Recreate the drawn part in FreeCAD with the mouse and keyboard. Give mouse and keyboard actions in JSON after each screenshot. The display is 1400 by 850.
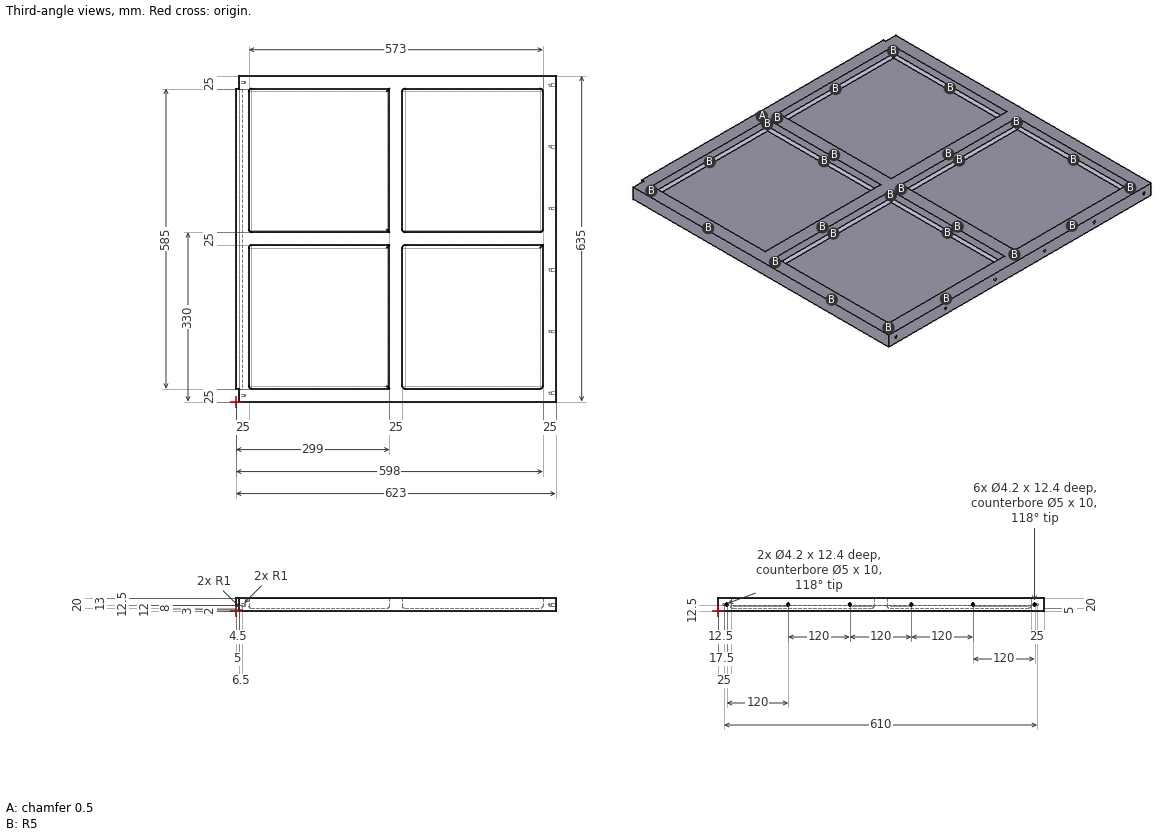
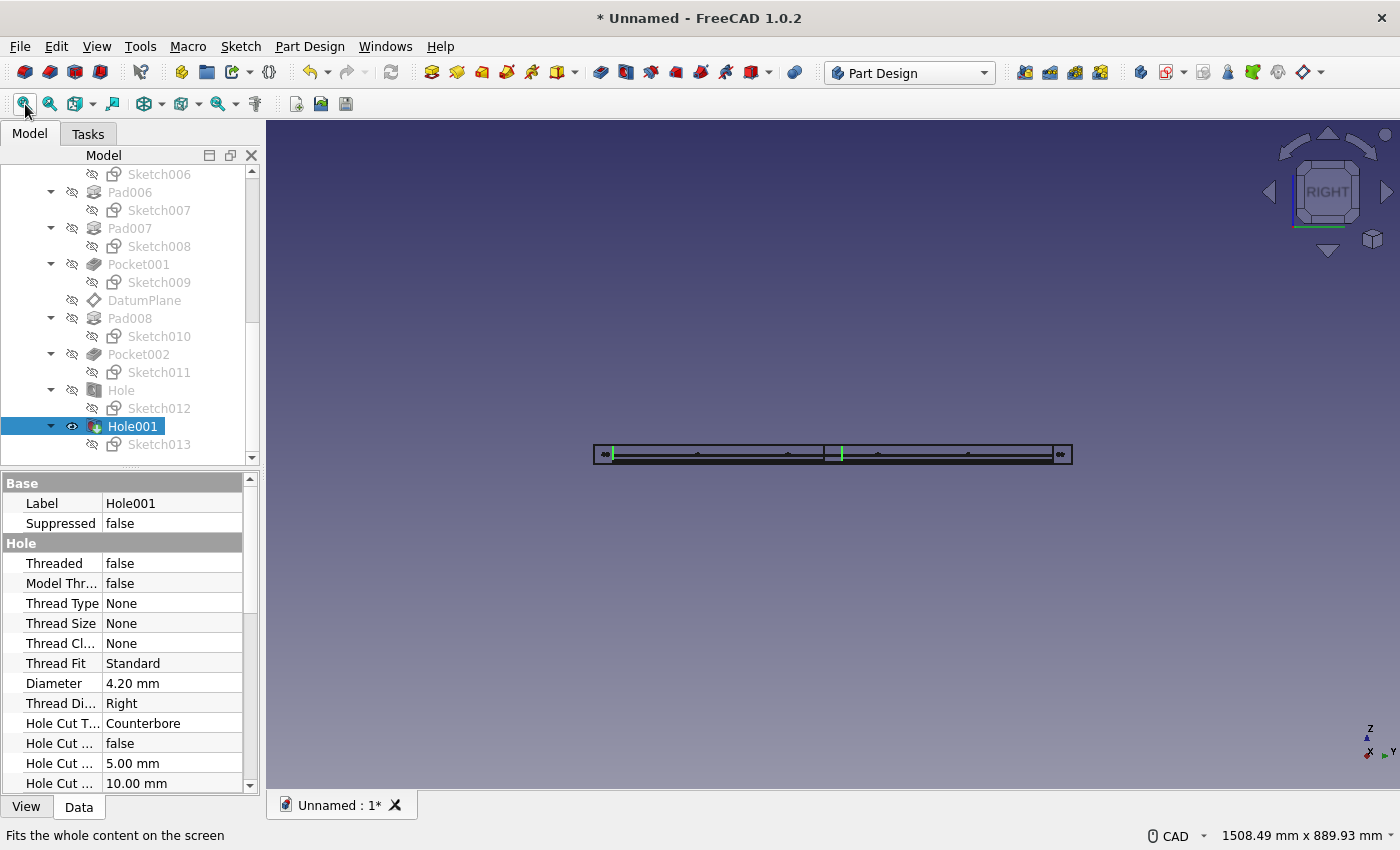
{"action": "left_click", "coordinate": [25, 104]}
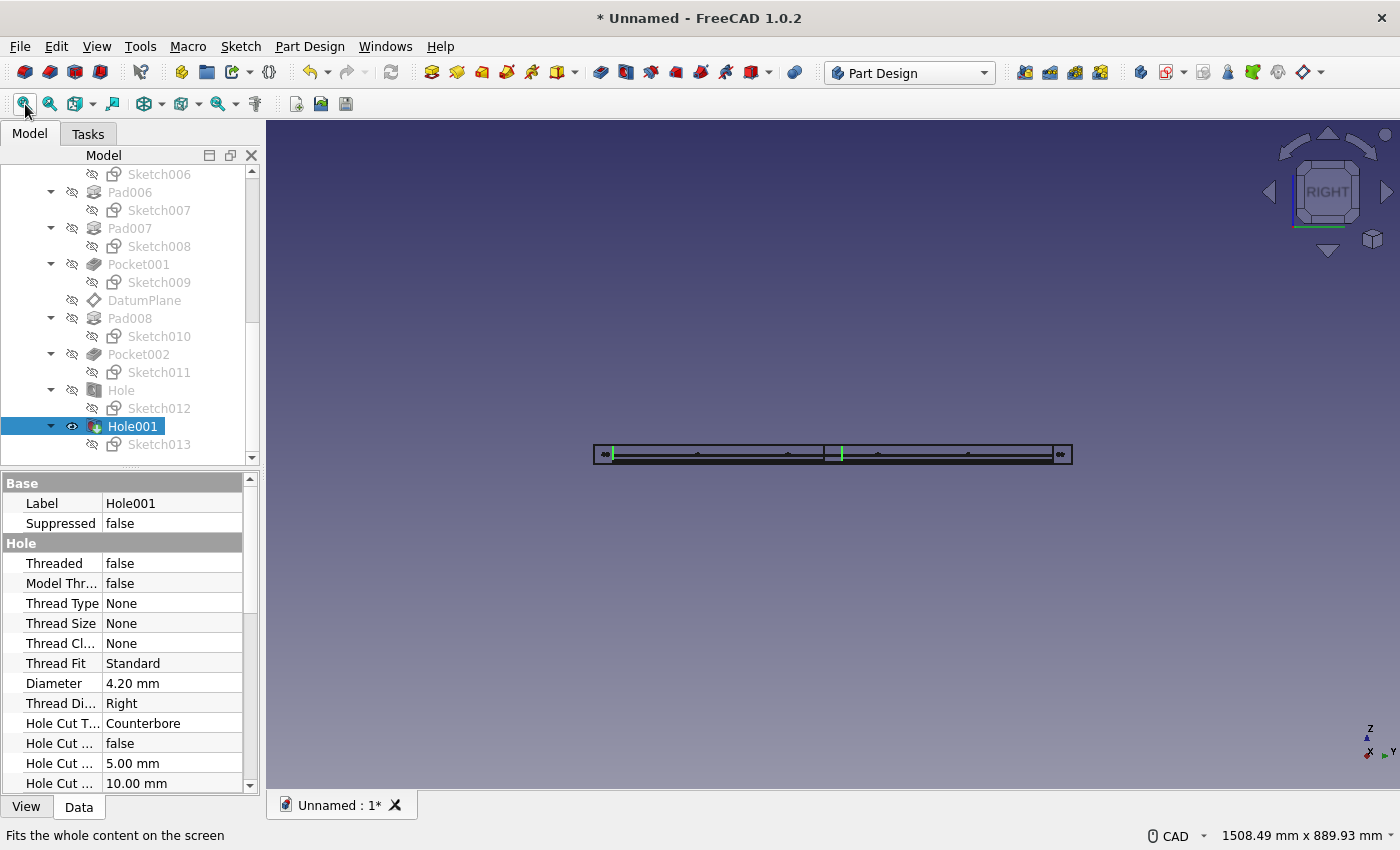
{"action": "scroll", "coordinate": [1053, 452], "scroll_direction": "up", "scroll_amount": 6}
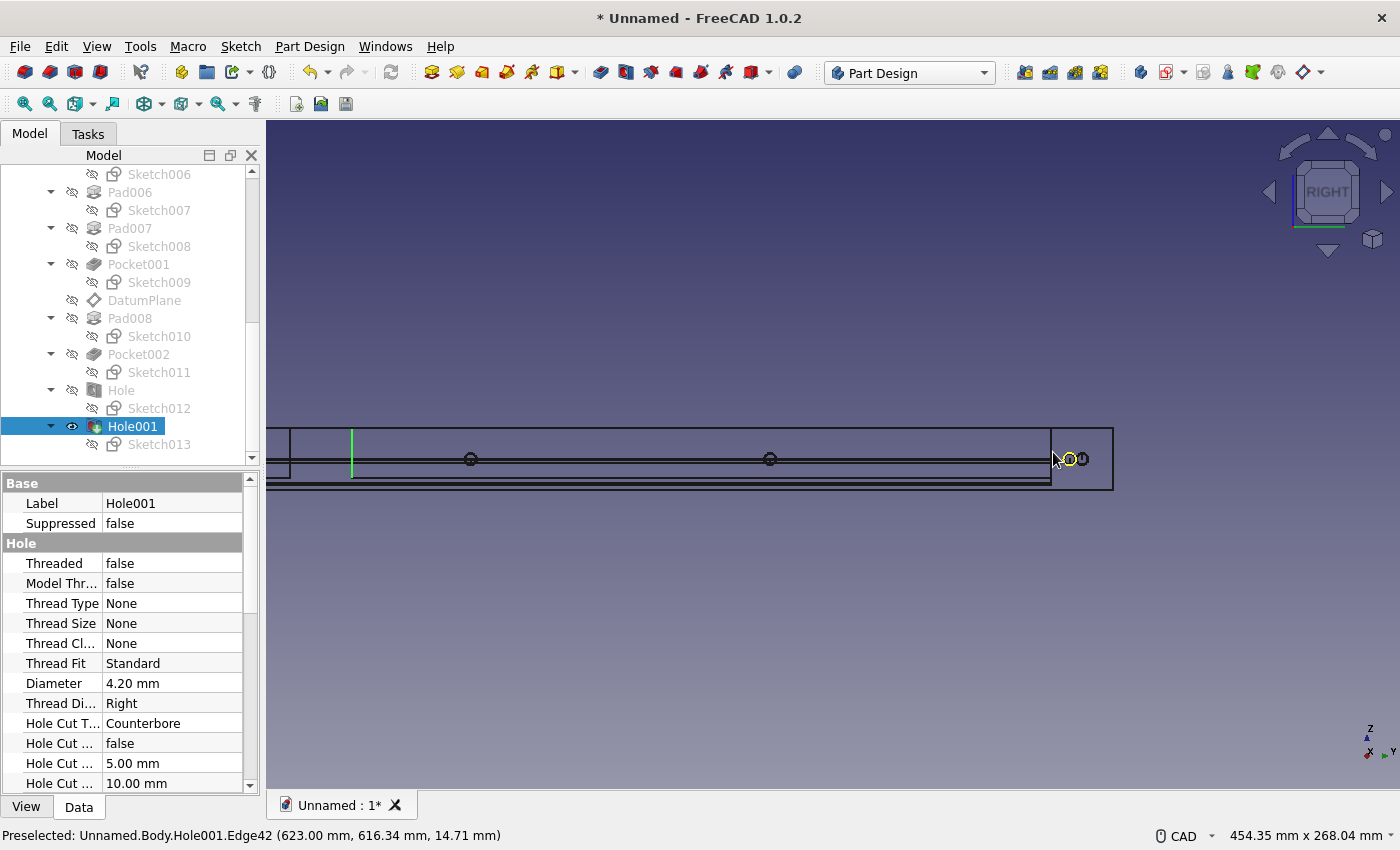
{"action": "left_click", "coordinate": [1051, 452], "text": "ctrl"}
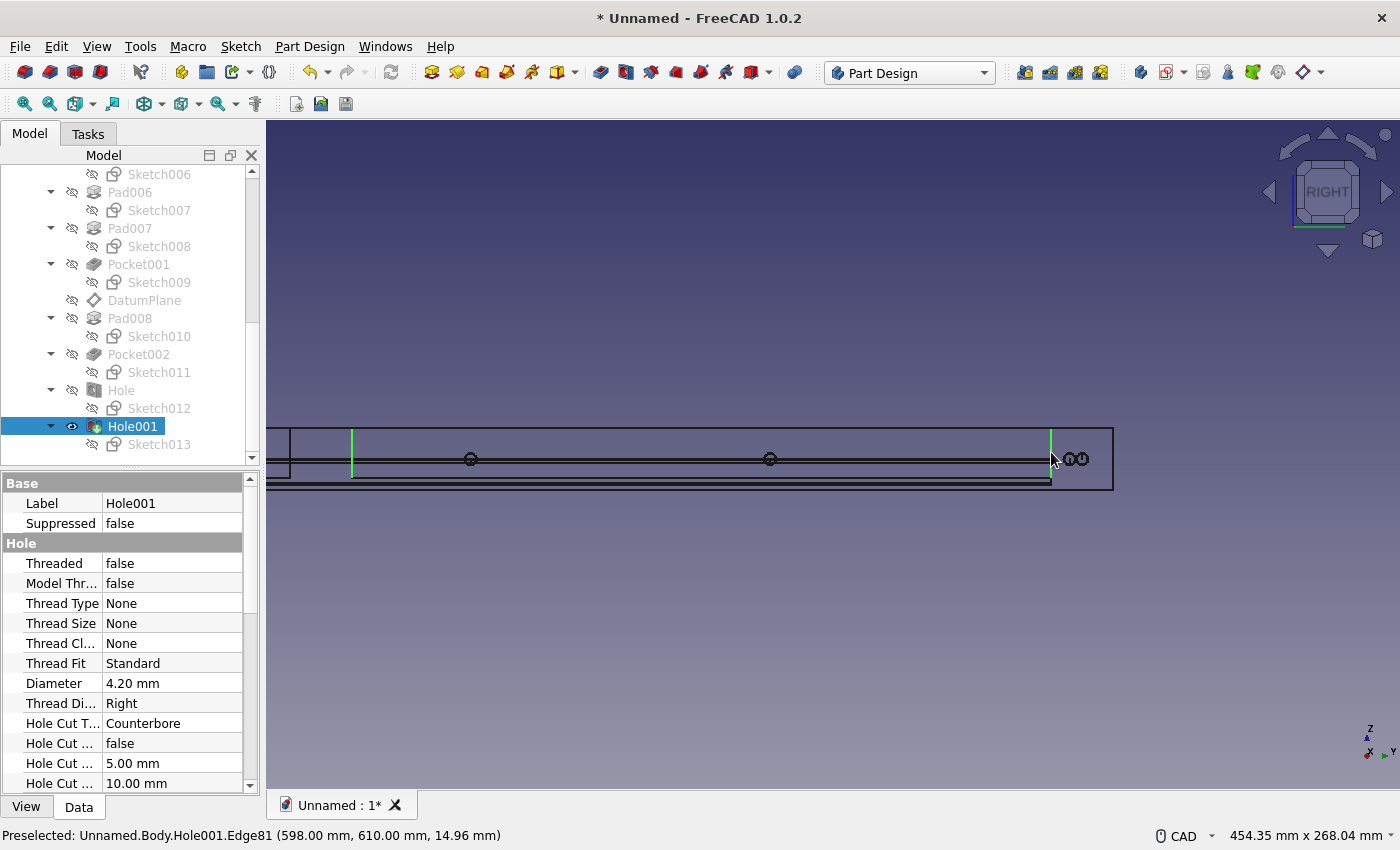
{"action": "key", "text": "v 1"}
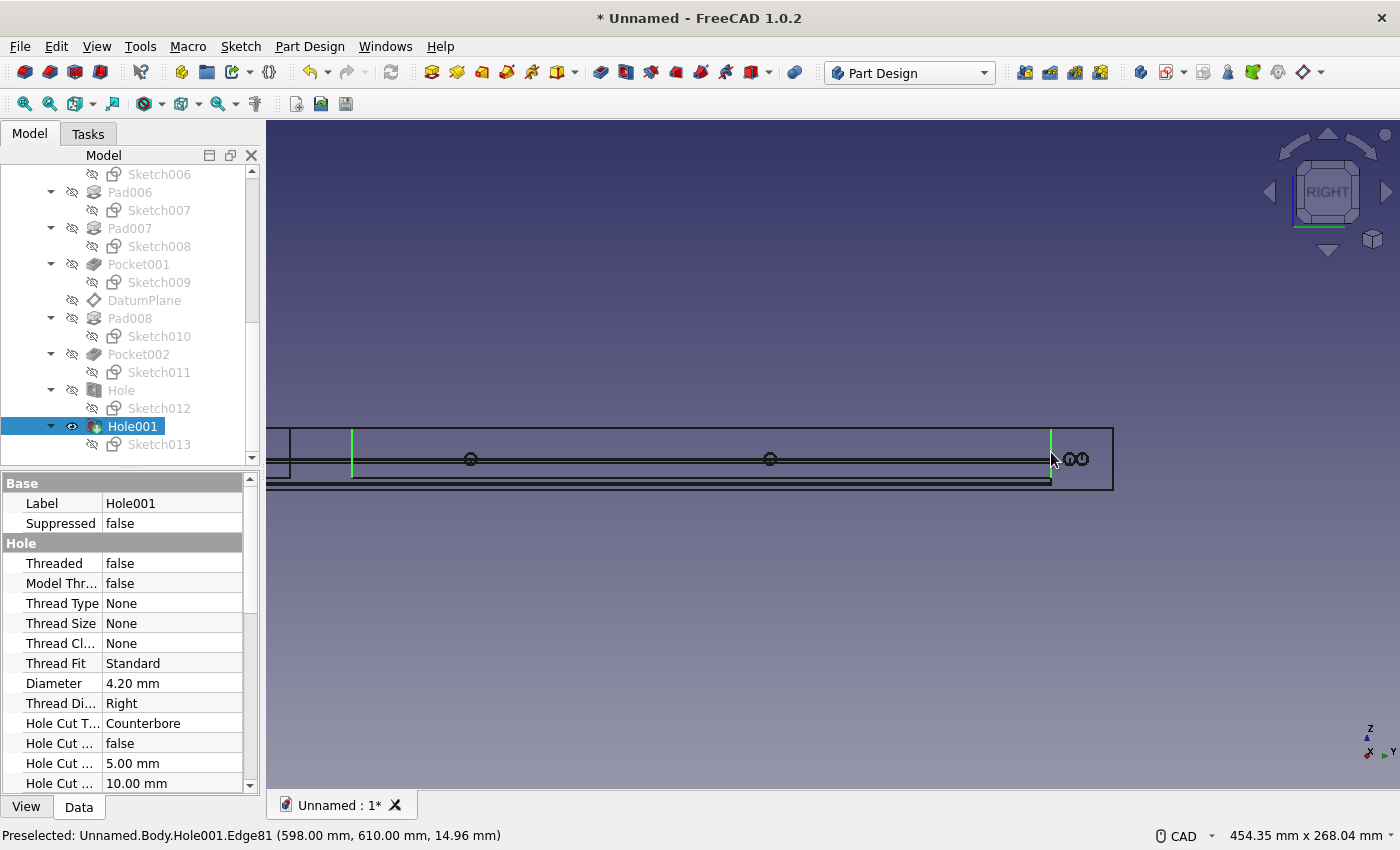
{"action": "left_click", "coordinate": [25, 72]}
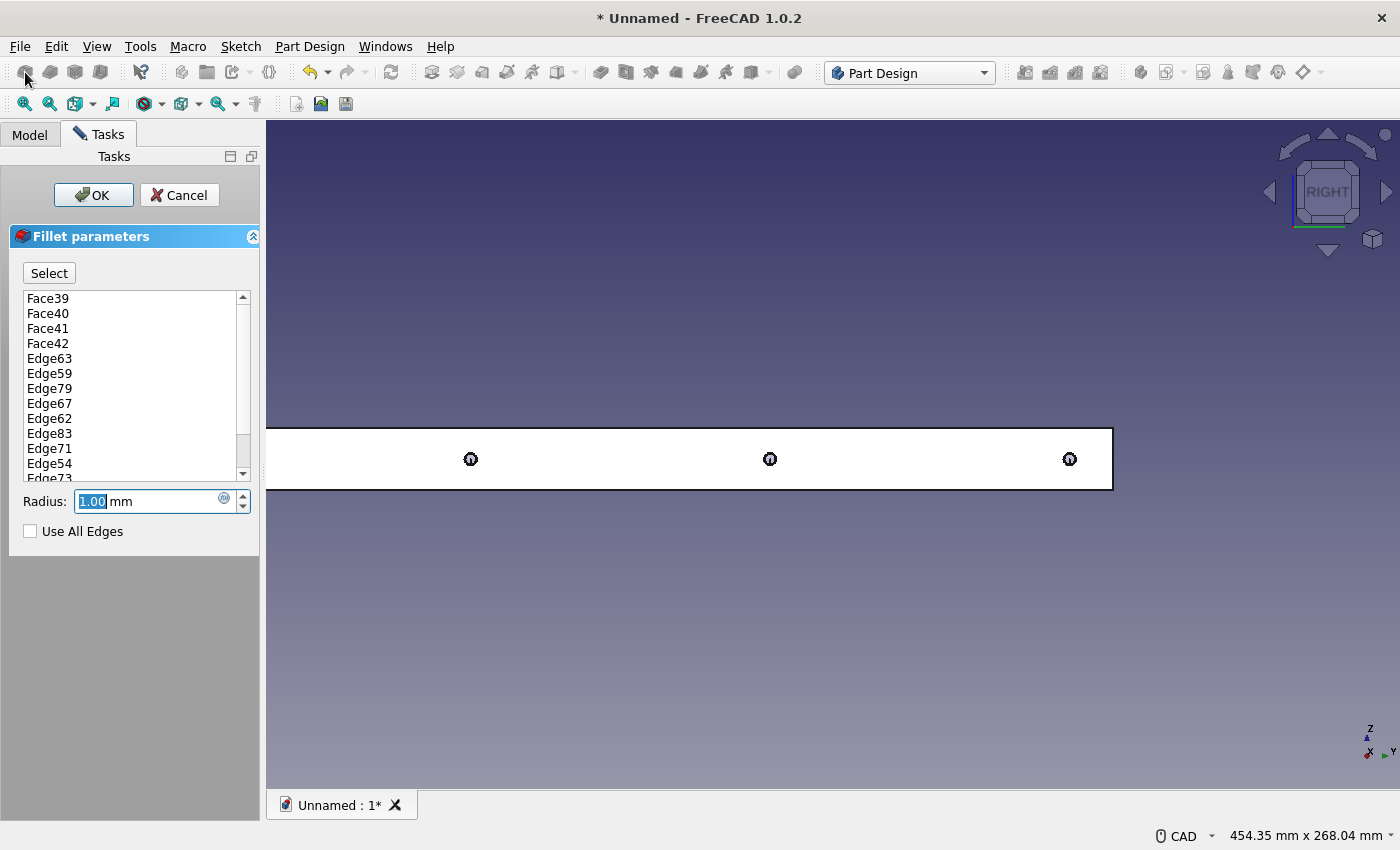
{"action": "type", "text": "5"}
{"action": "key", "text": "Tab"}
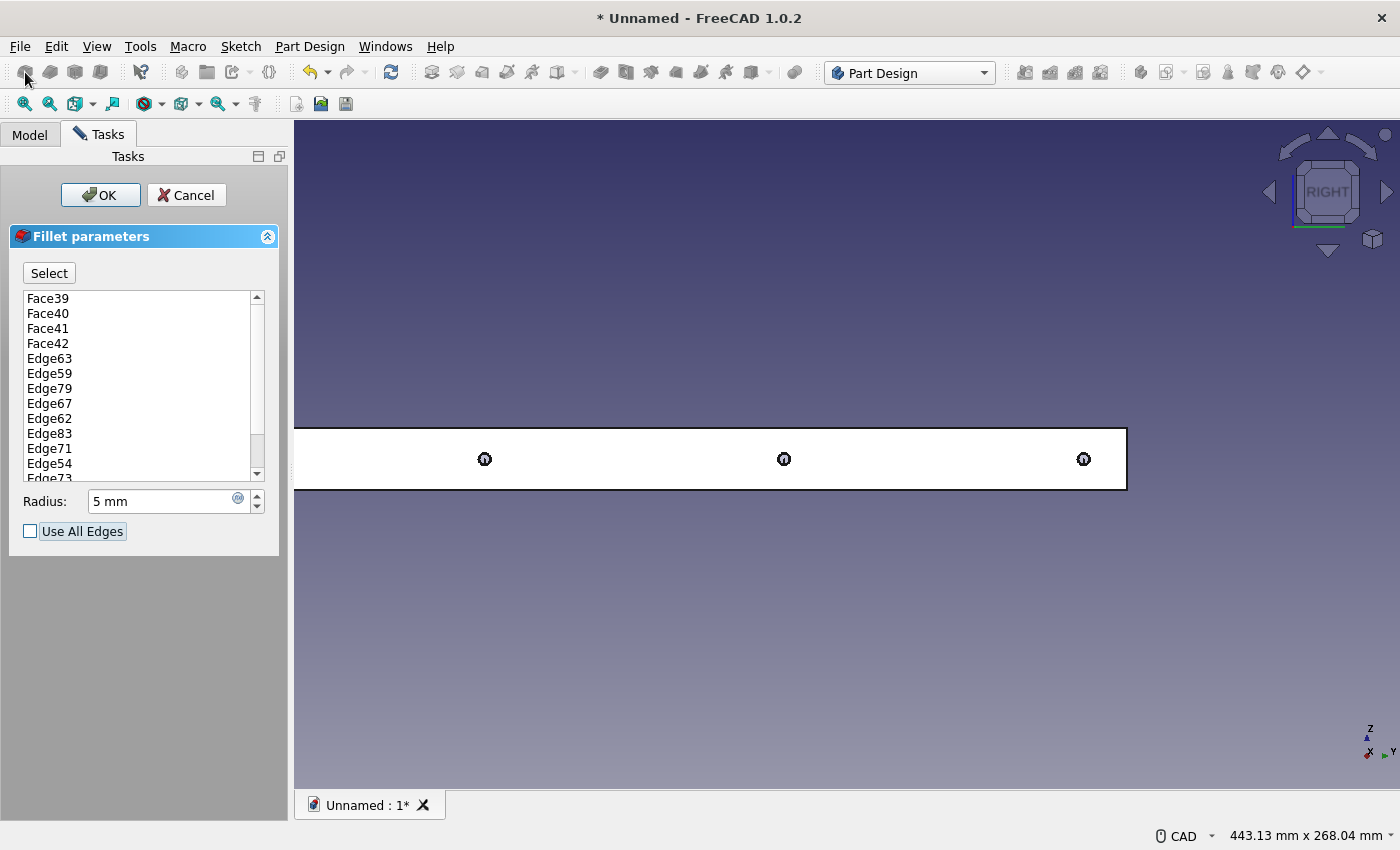
{"action": "left_click", "coordinate": [101, 195]}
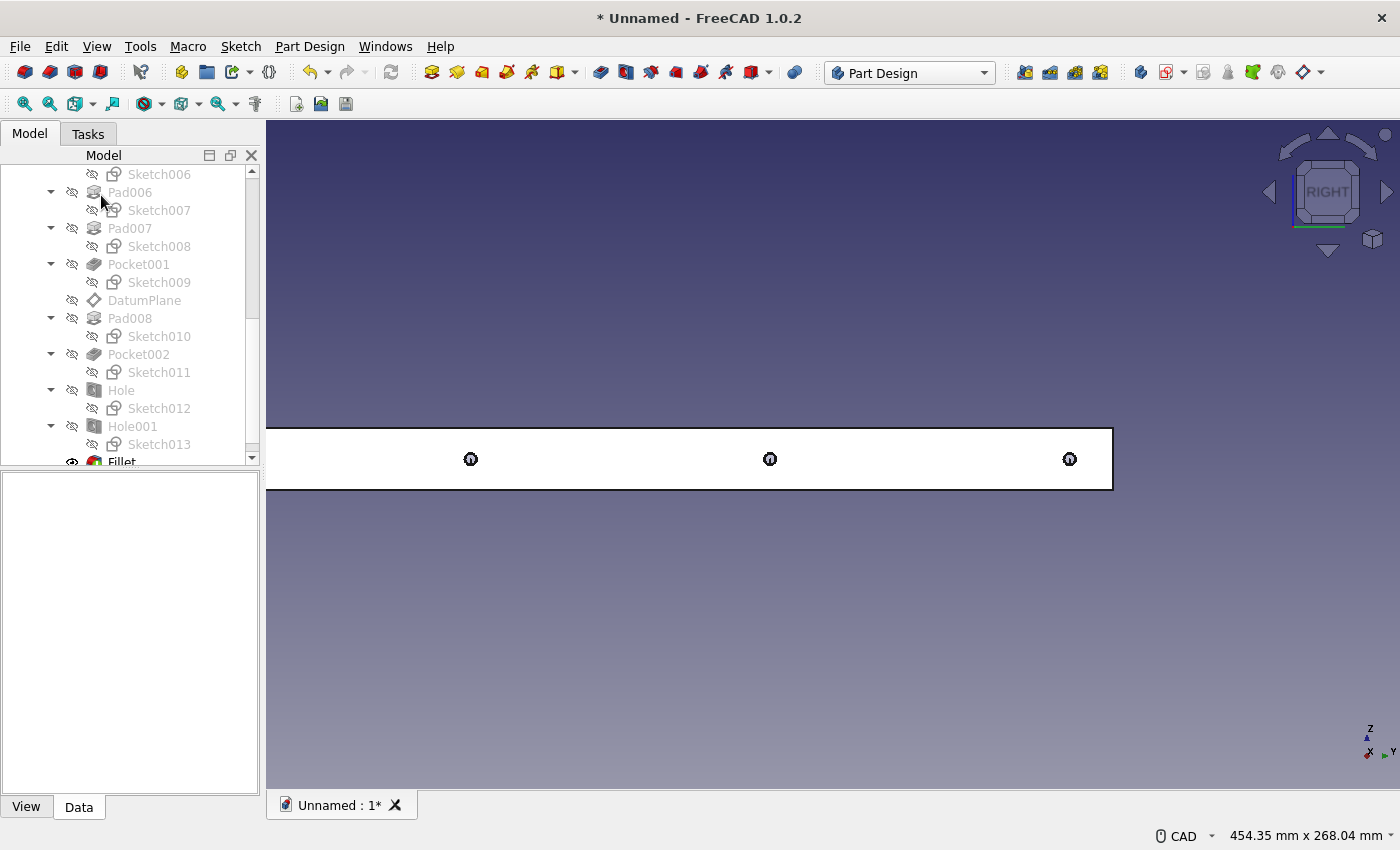
{"action": "key", "text": "0"}